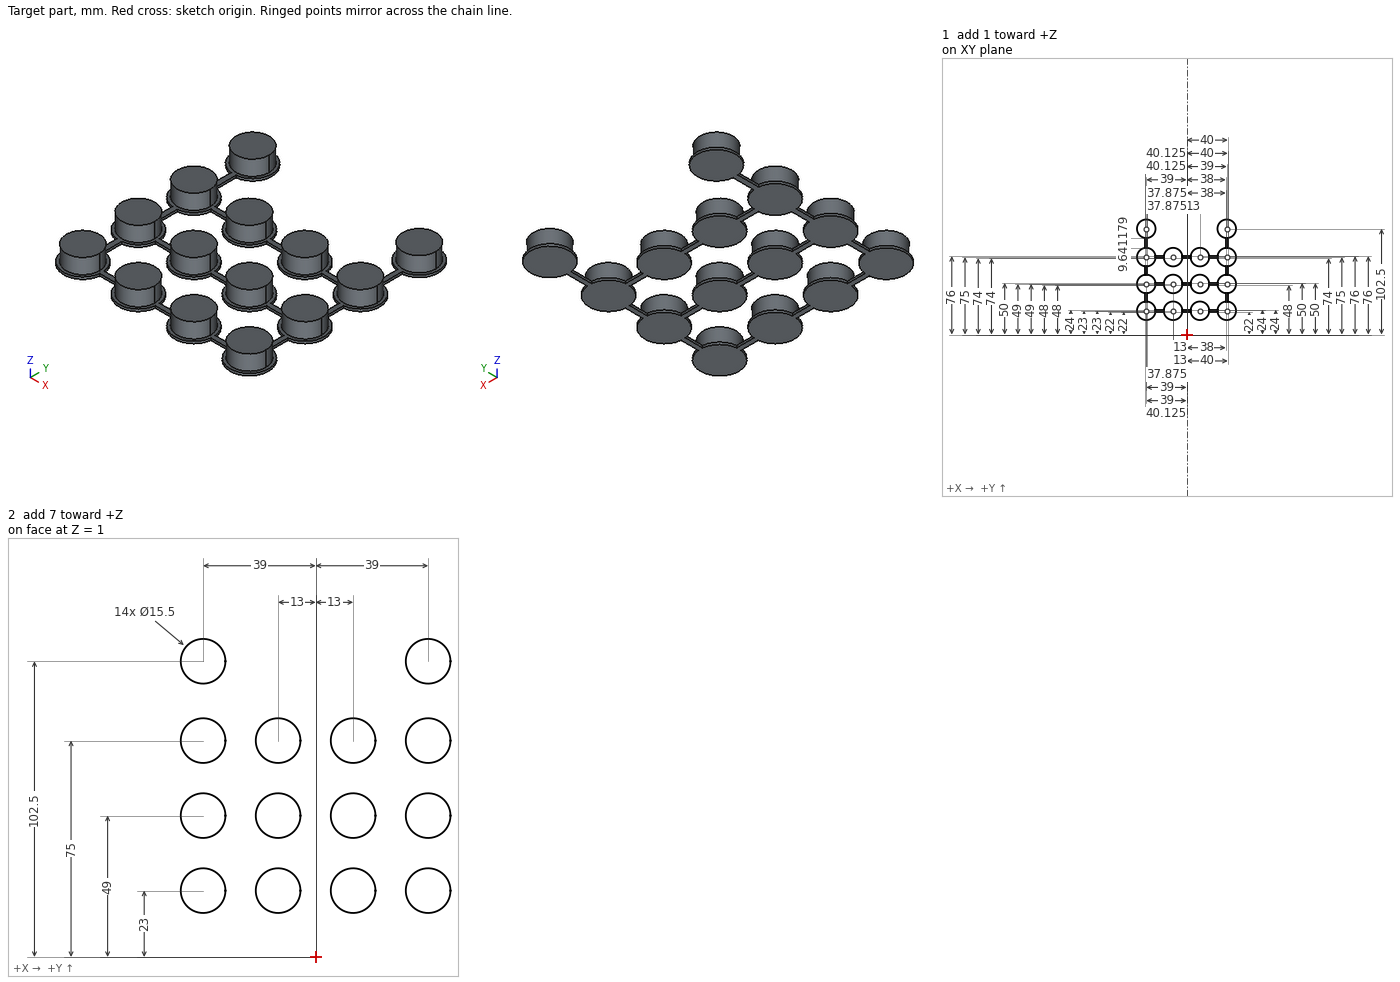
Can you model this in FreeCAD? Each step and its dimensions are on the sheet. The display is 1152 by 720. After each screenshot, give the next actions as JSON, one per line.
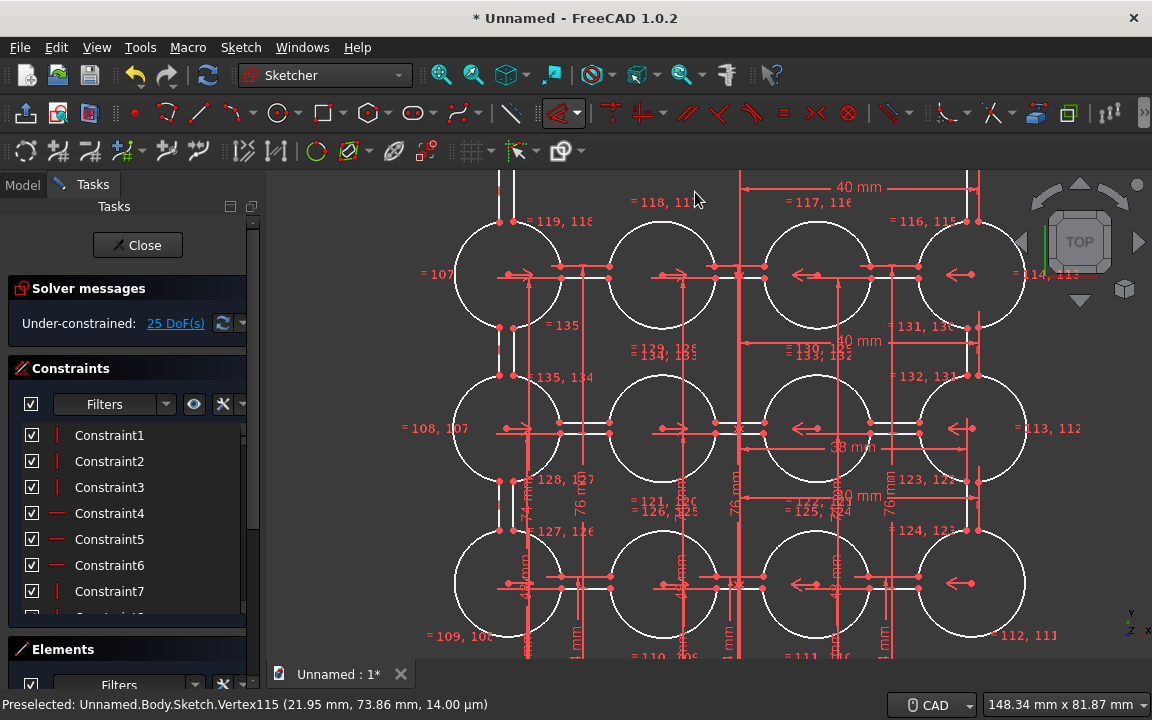
{"action": "left_click", "coordinate": [967, 328]}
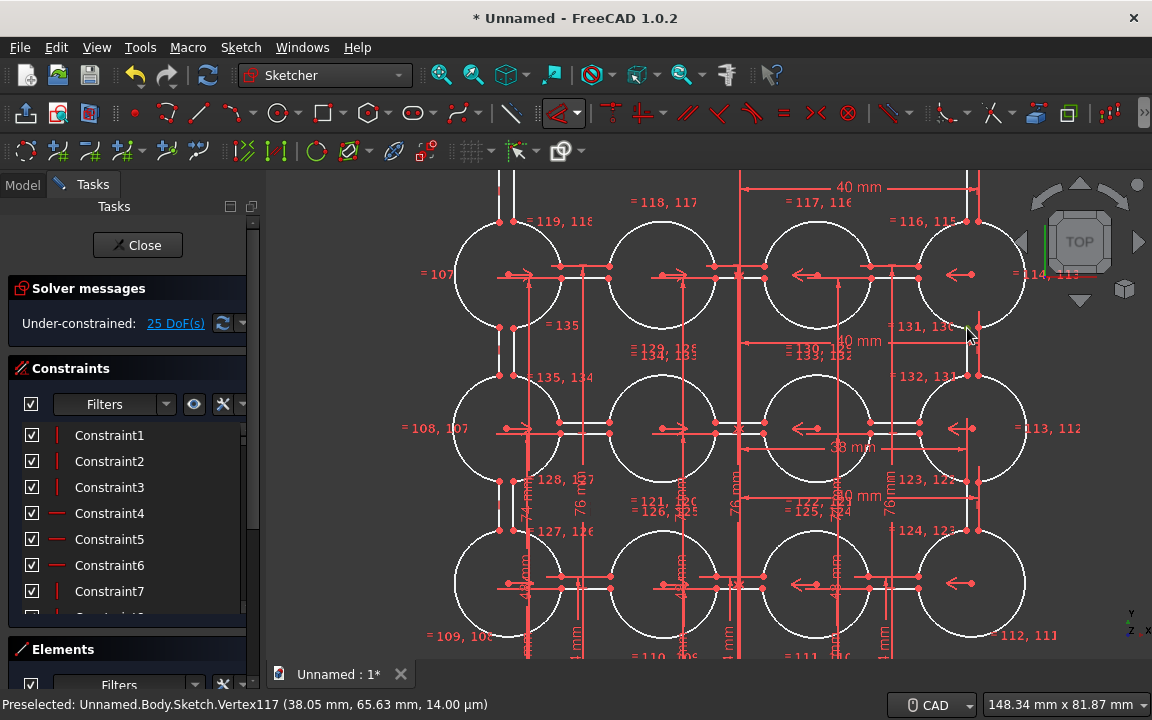
{"action": "key", "text": "l"}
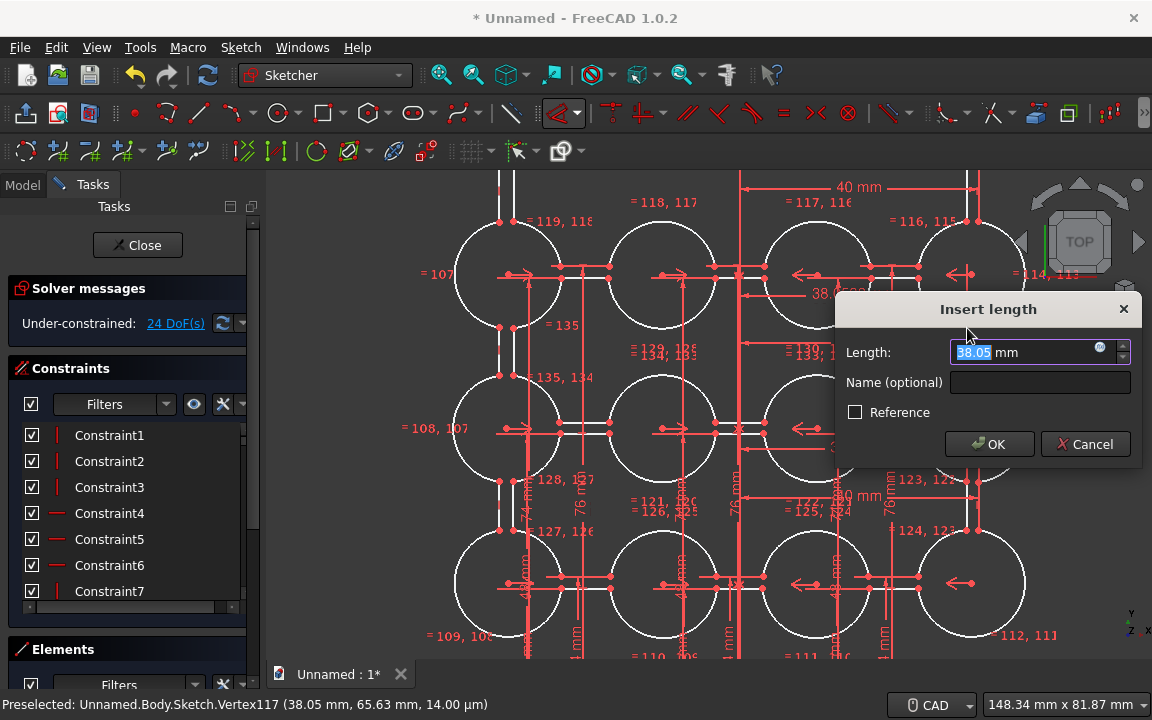
{"action": "type", "text": "38"}
{"action": "key", "text": "Return"}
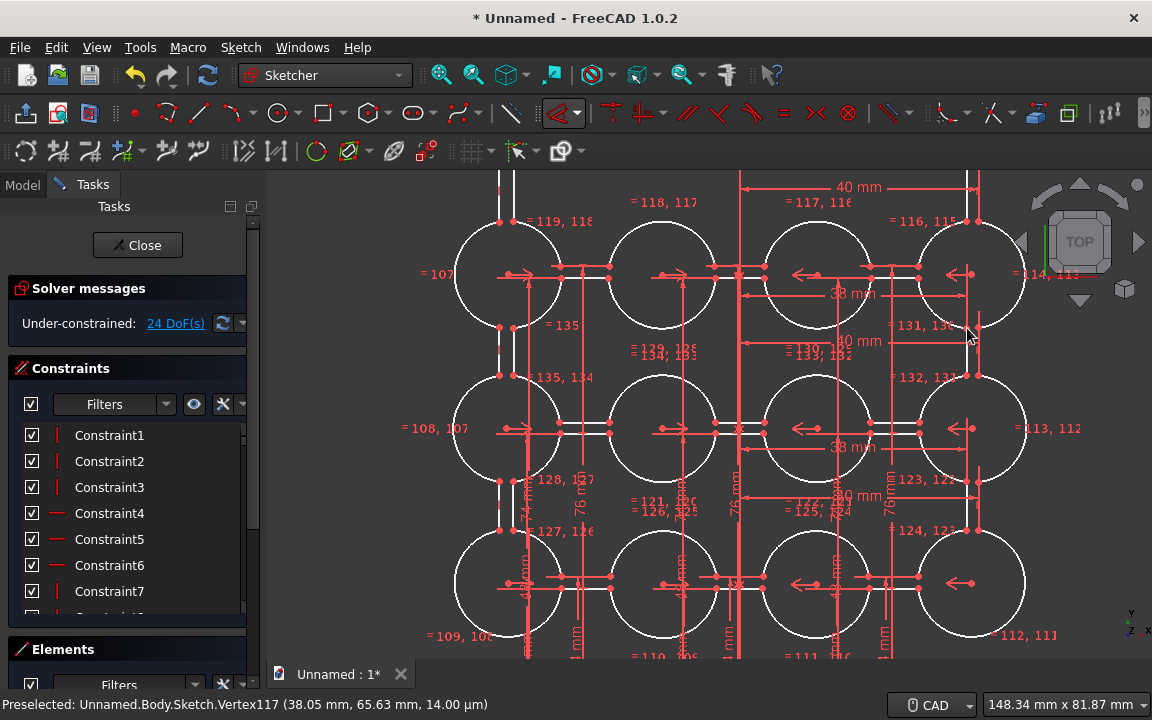
{"action": "left_click", "coordinate": [920, 423]}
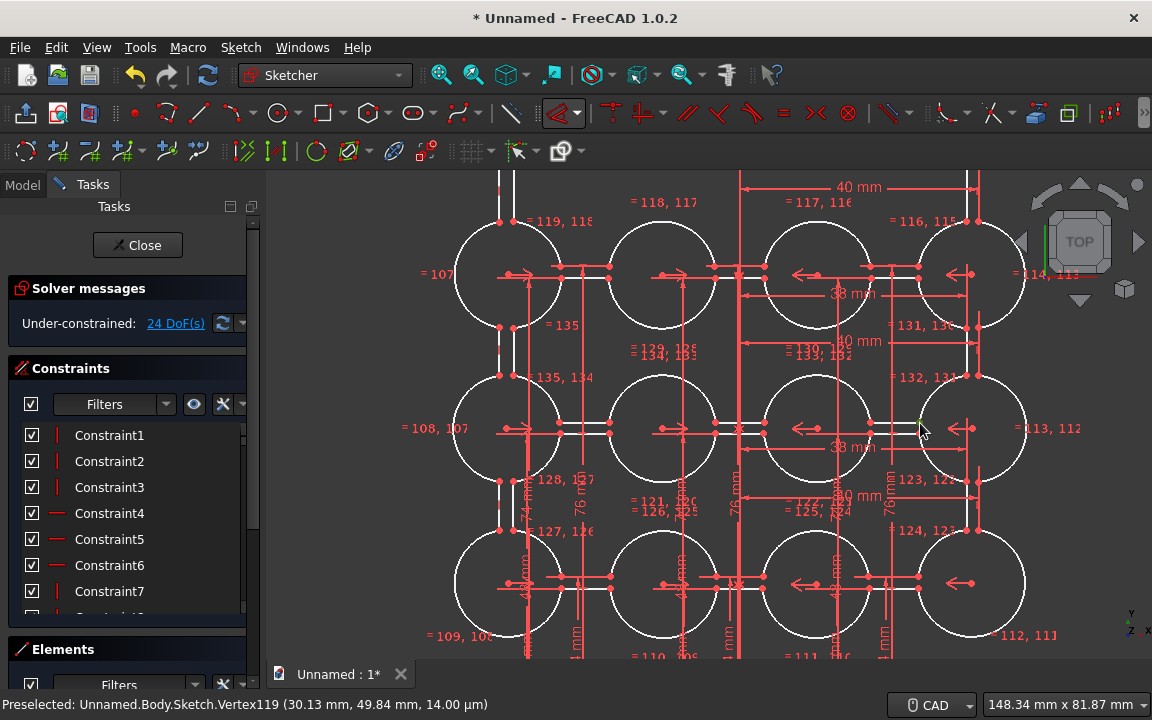
{"action": "left_click", "coordinate": [580, 114]}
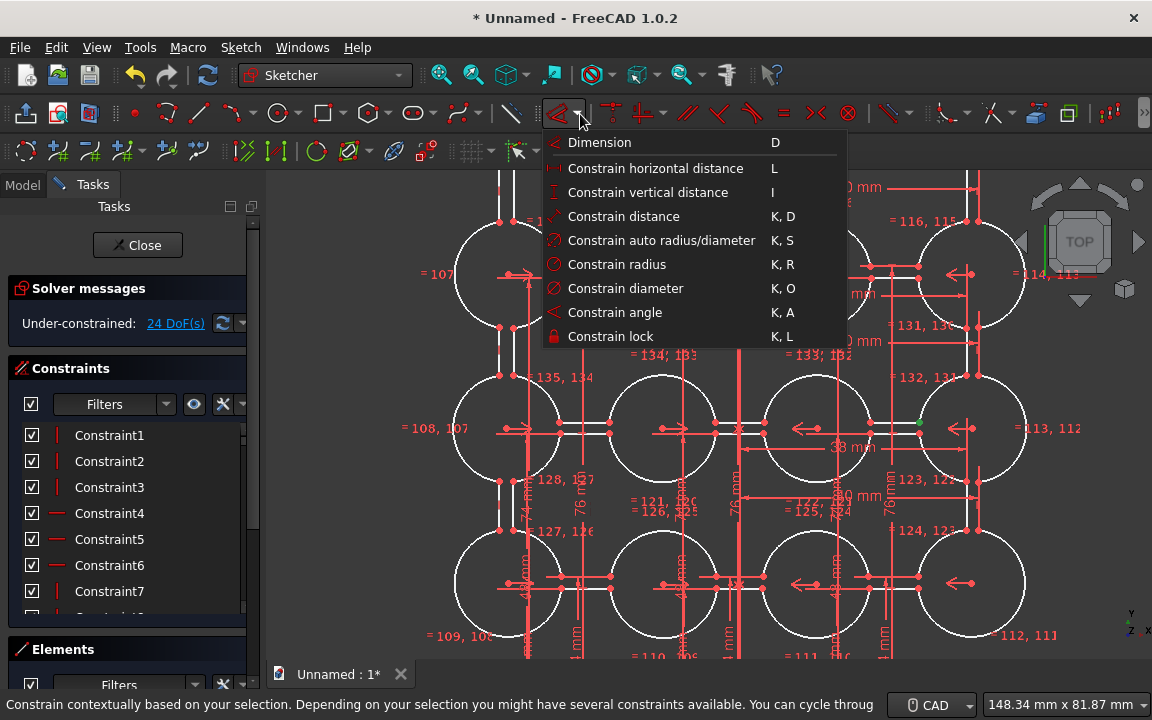
{"action": "left_click", "coordinate": [695, 192]}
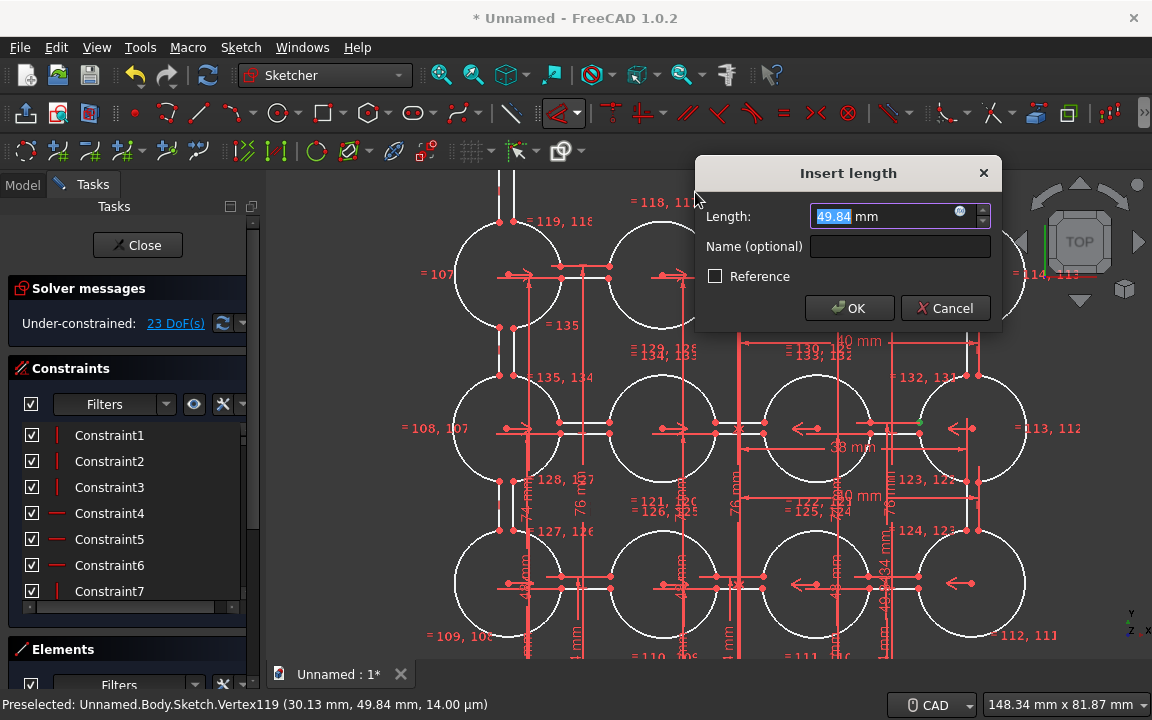
{"action": "type", "text": "50"}
{"action": "key", "text": "Return"}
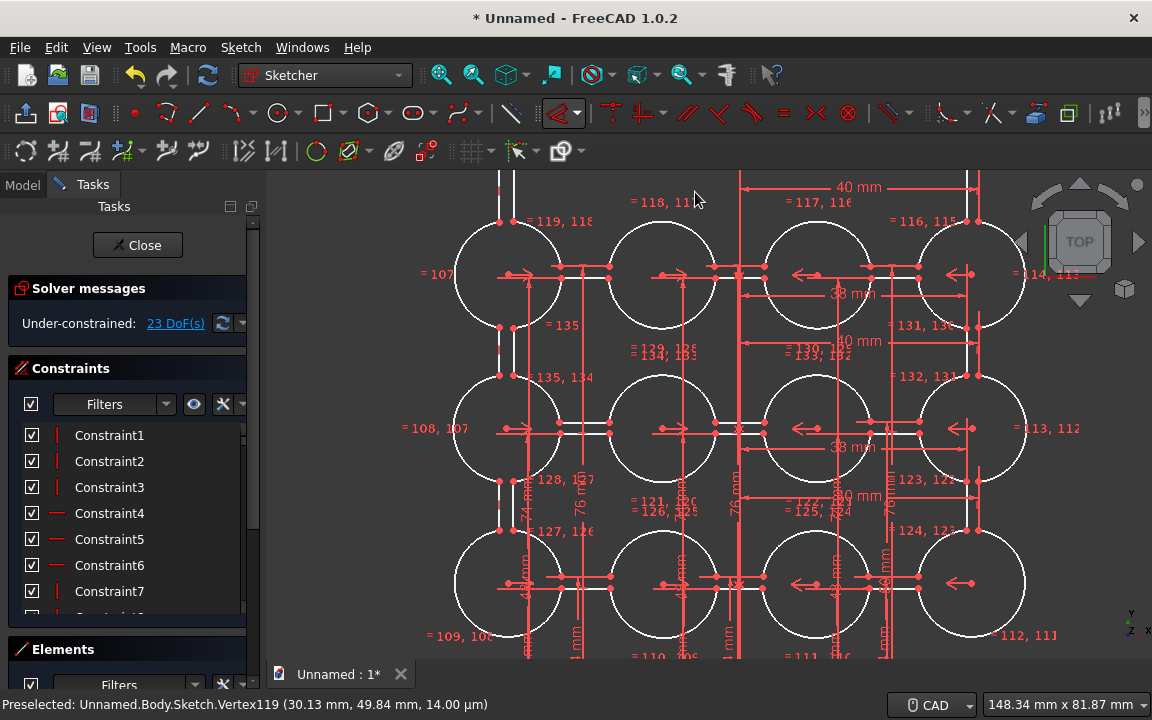
{"action": "left_click", "coordinate": [764, 423]}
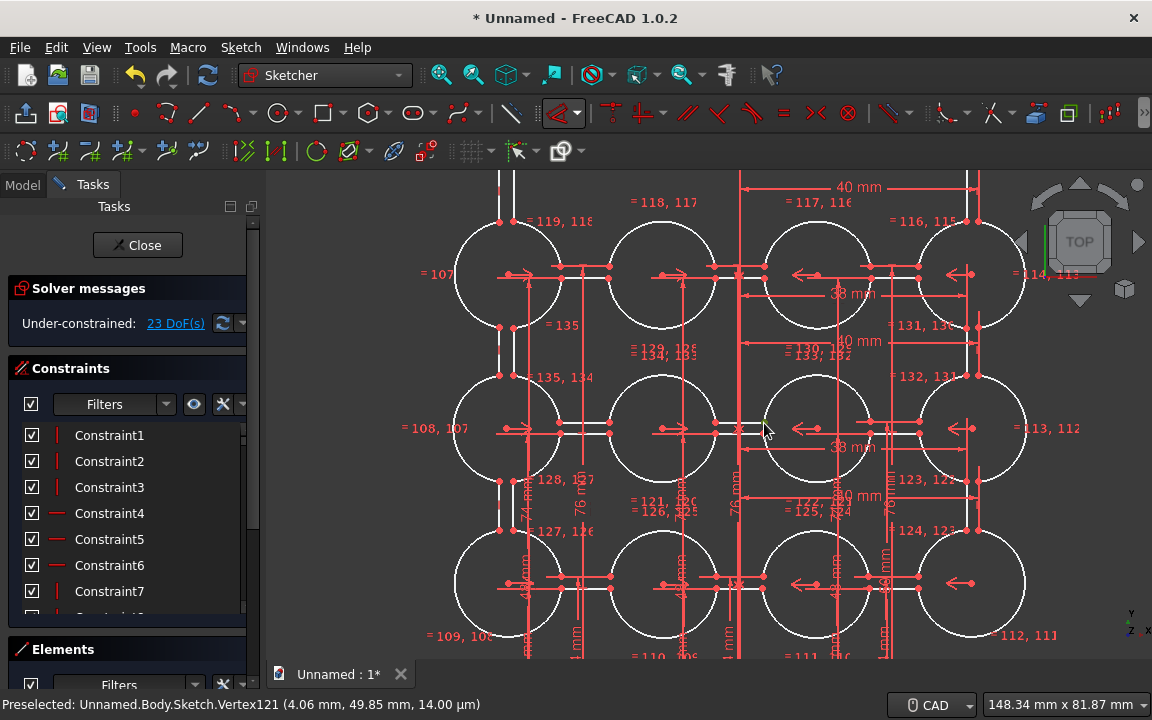
{"action": "key", "text": "i"}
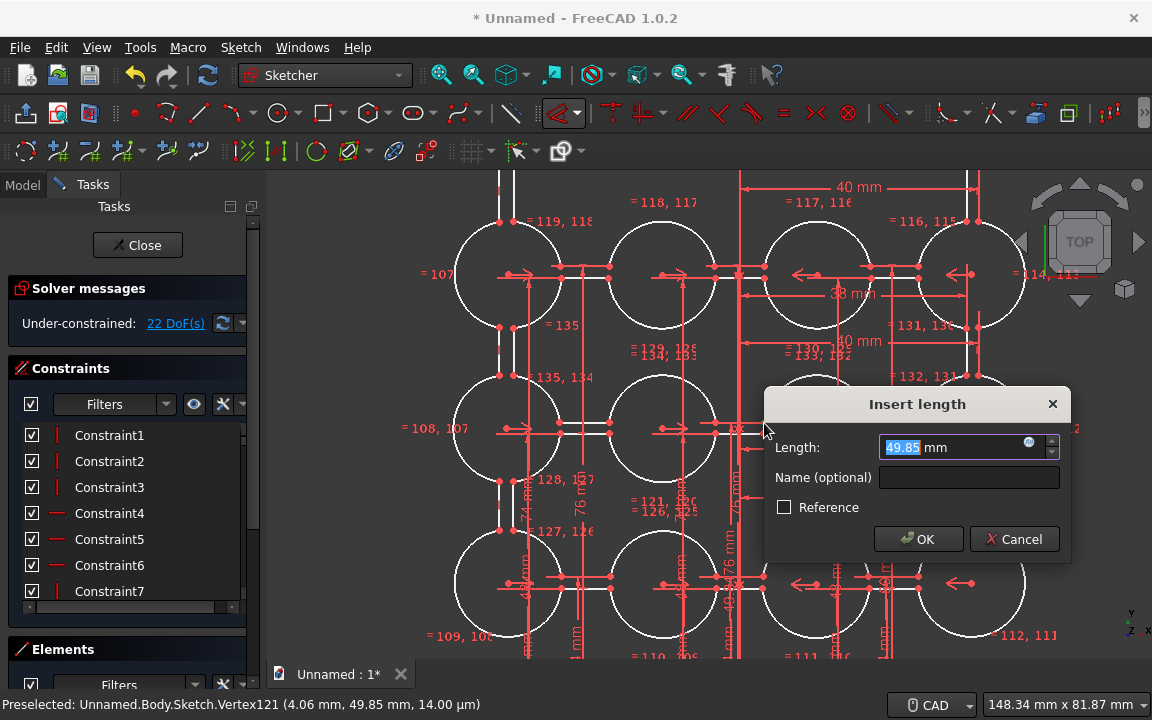
{"action": "type", "text": "50"}
{"action": "key", "text": "Return"}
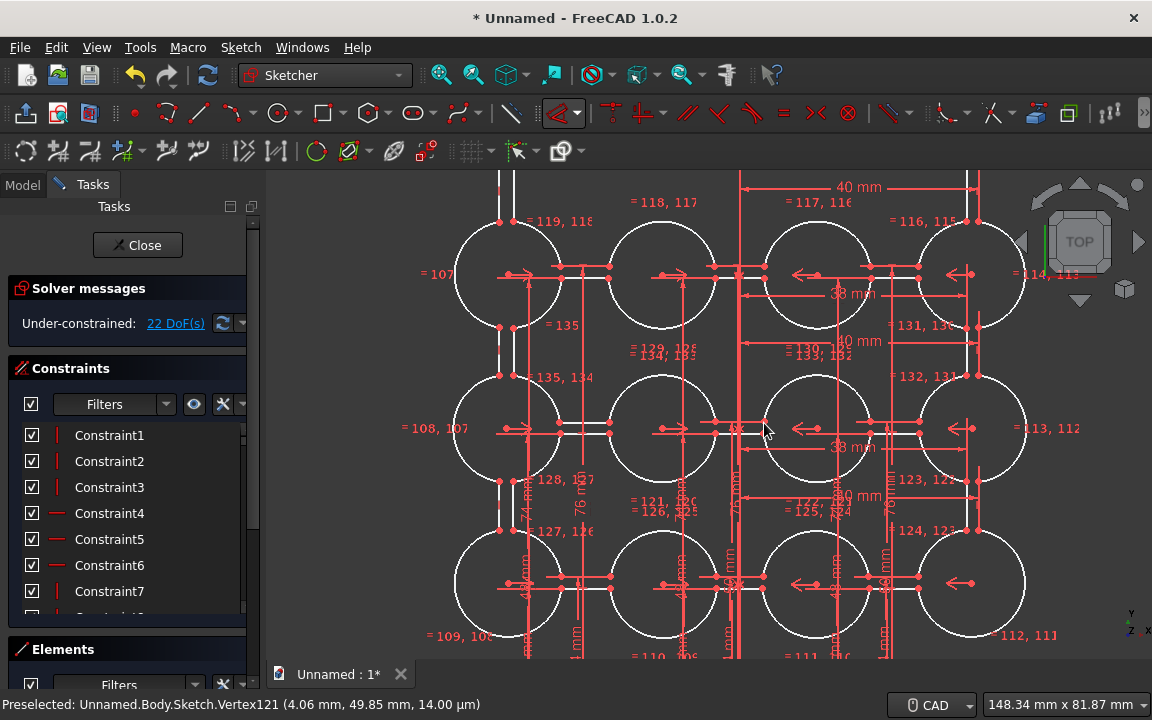
{"action": "left_click", "coordinate": [609, 423]}